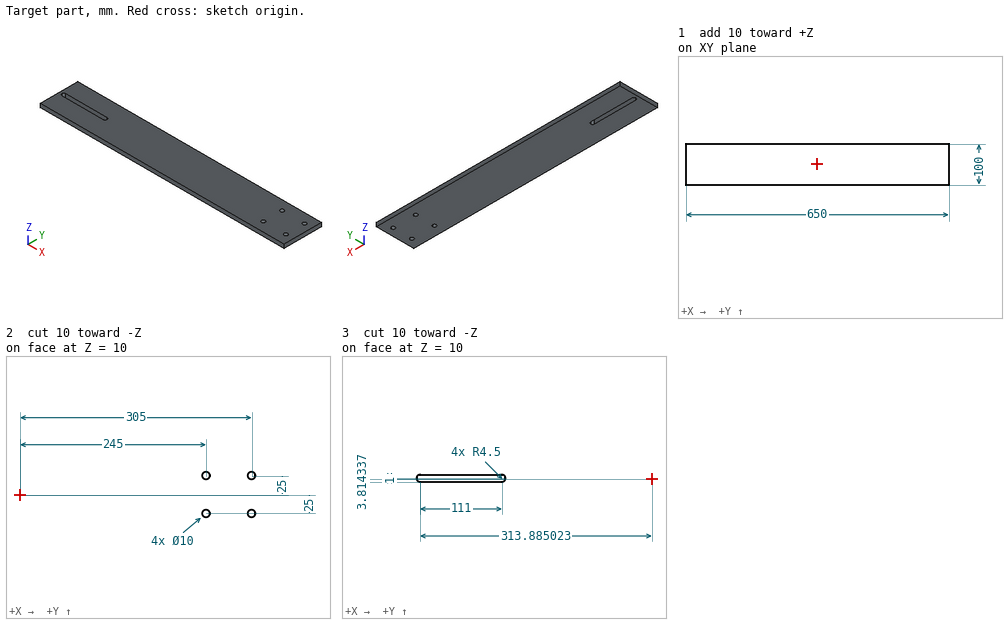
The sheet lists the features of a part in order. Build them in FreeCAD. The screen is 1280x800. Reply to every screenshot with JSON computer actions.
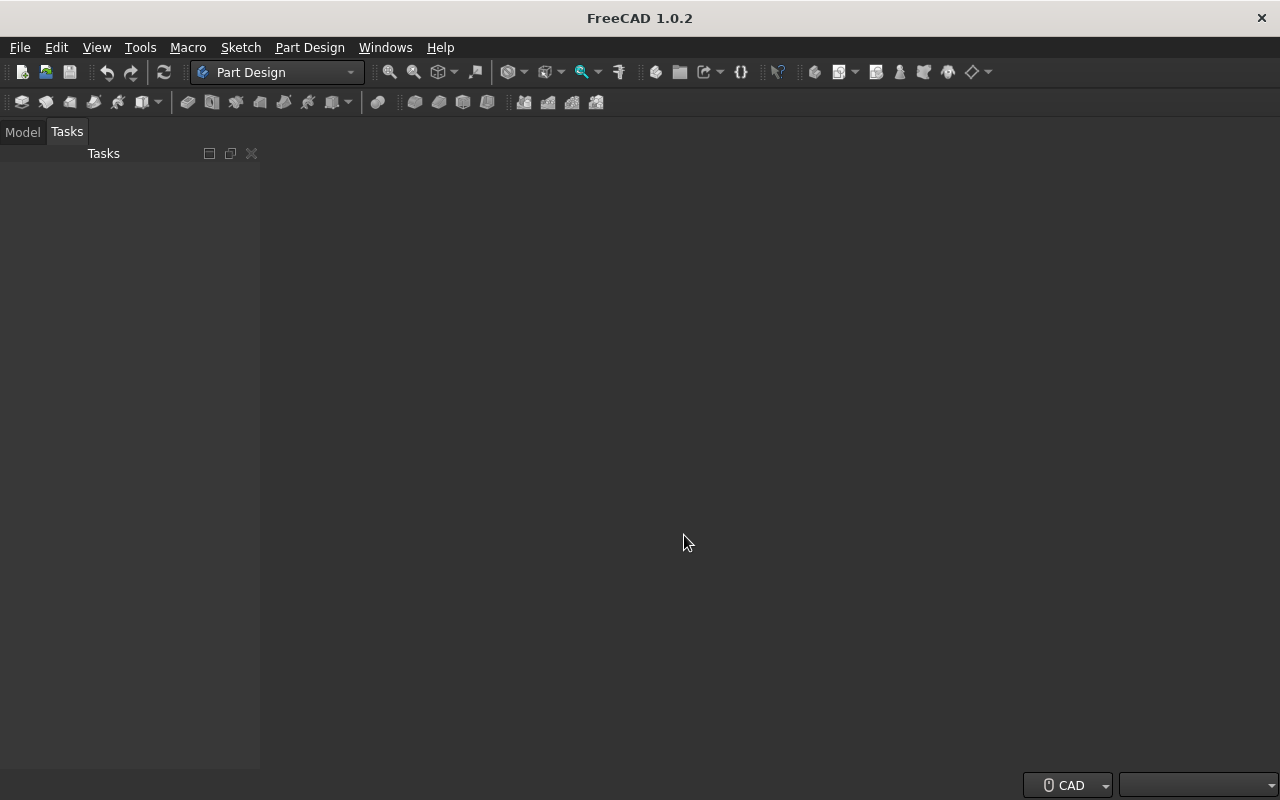
{"action": "key", "text": "ctrl+n"}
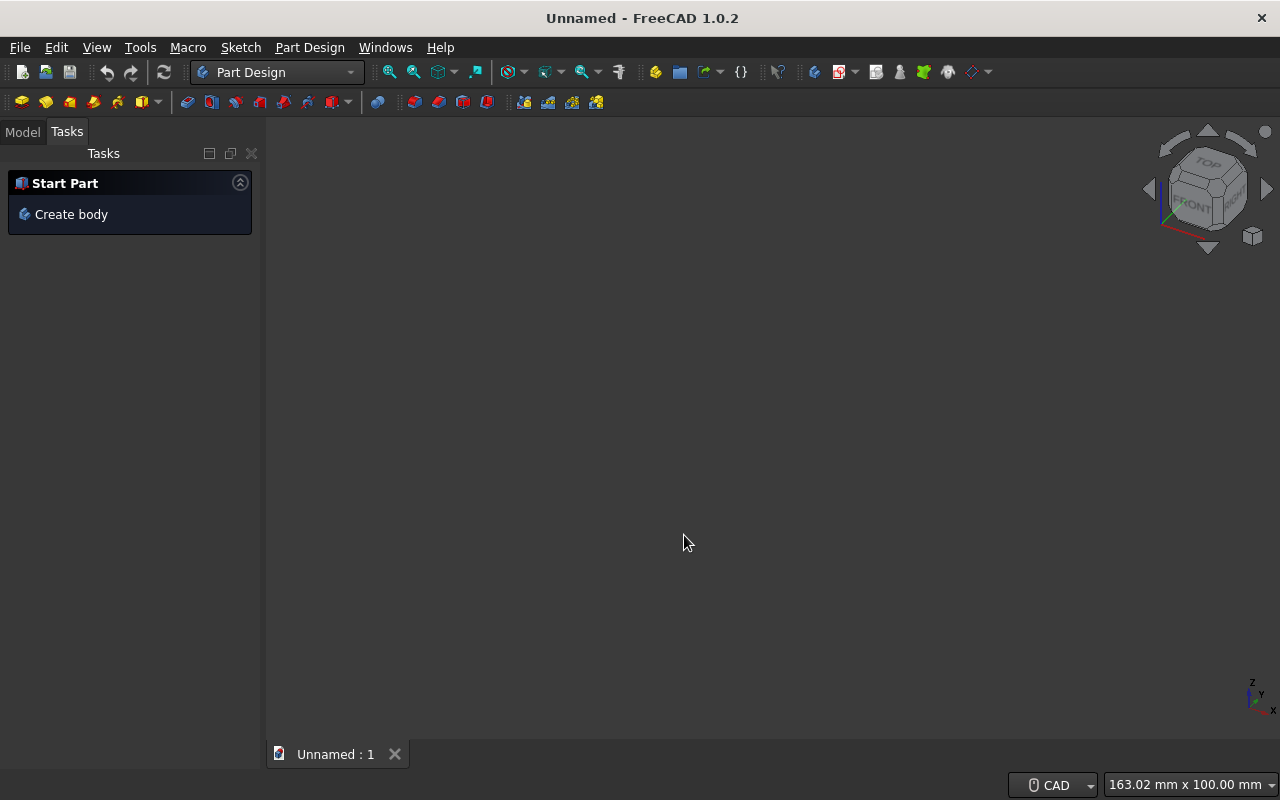
{"action": "left_click", "coordinate": [840, 72]}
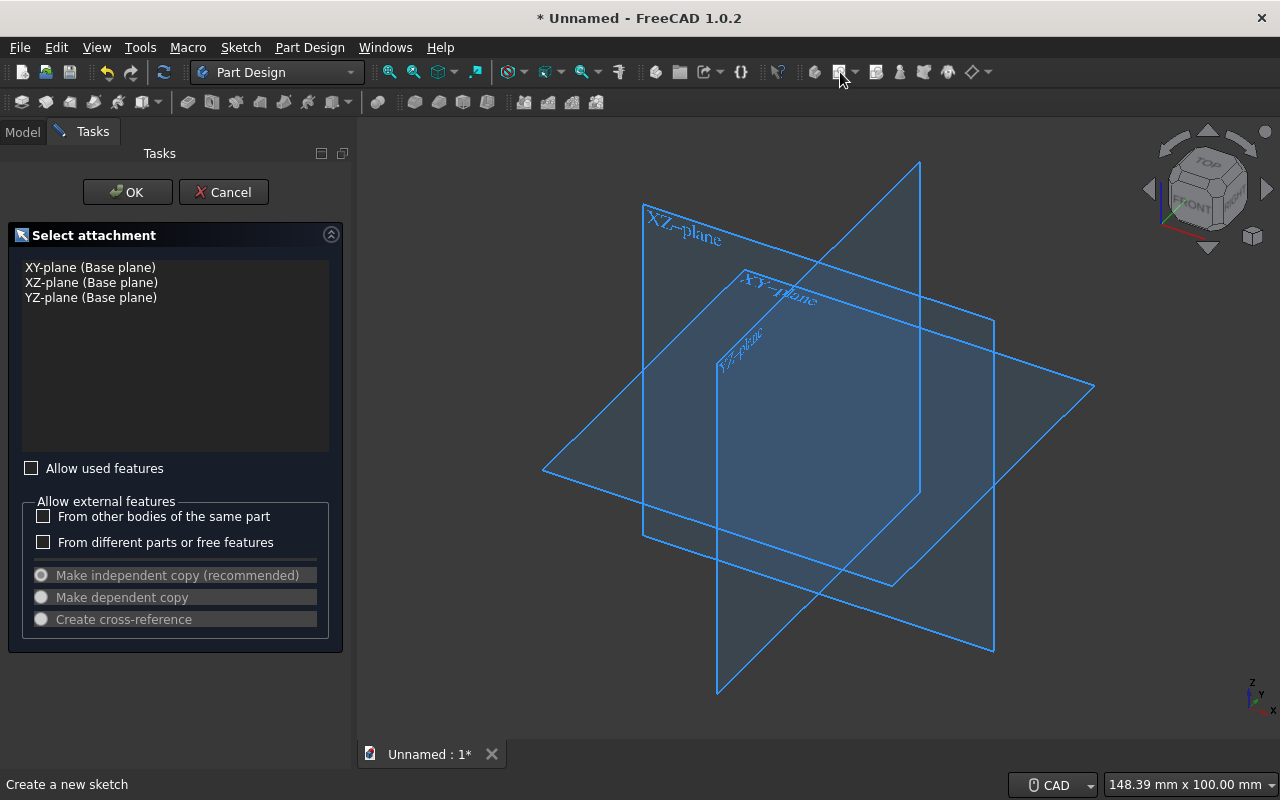
{"action": "left_click", "coordinate": [82, 268]}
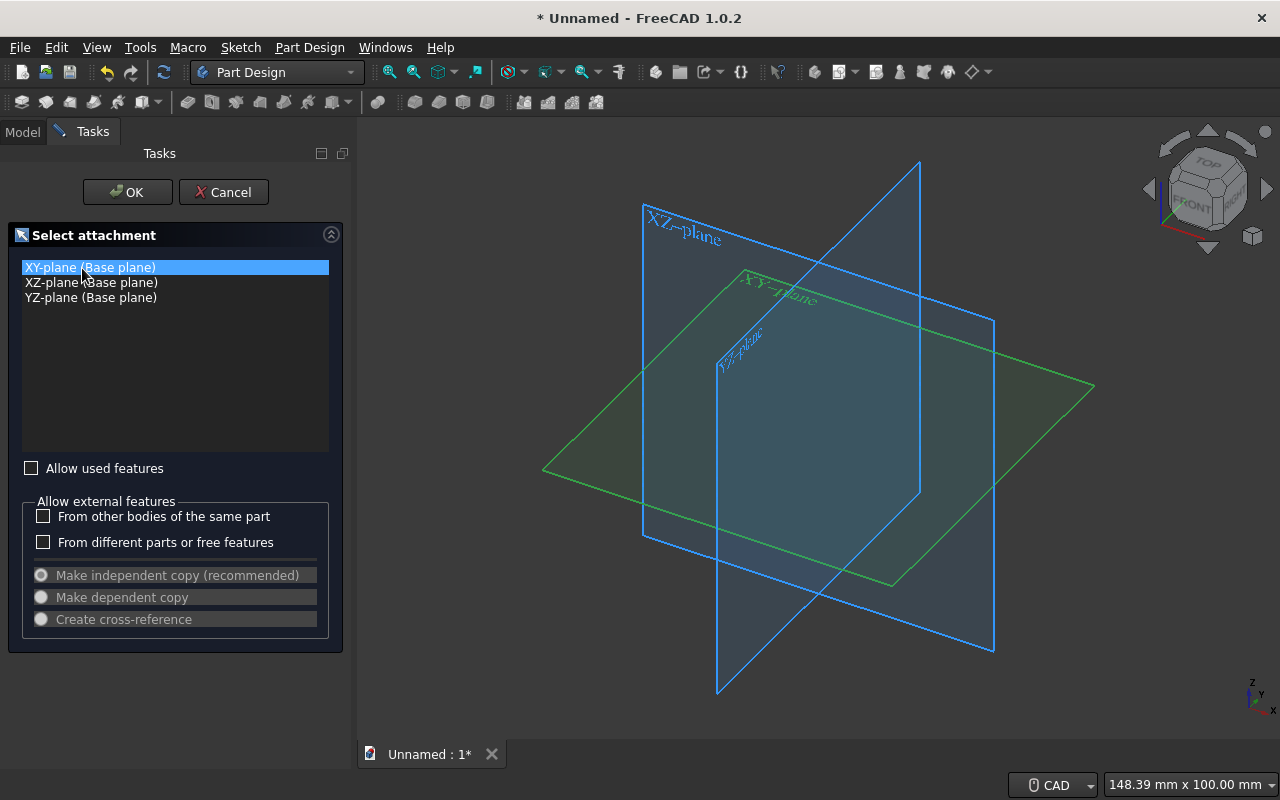
{"action": "left_click", "coordinate": [128, 192]}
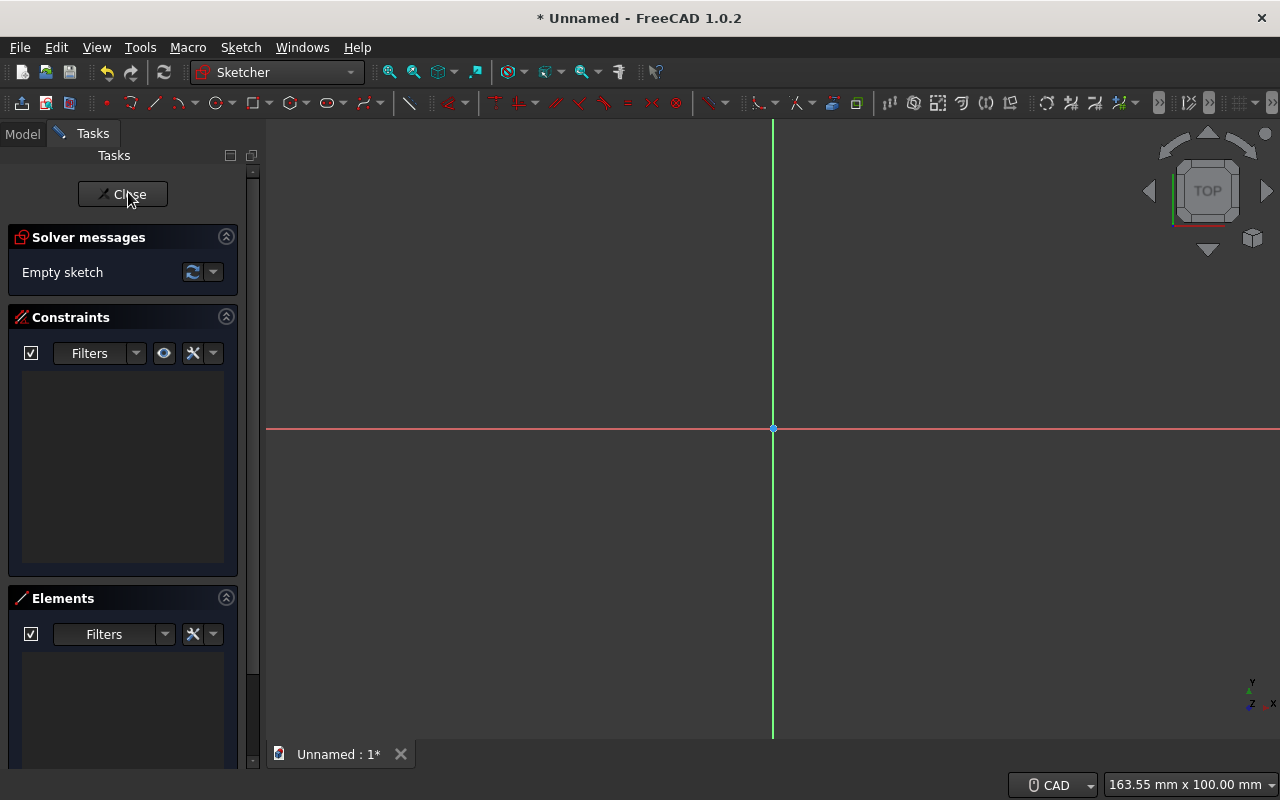
{"action": "scroll", "coordinate": [694, 429], "scroll_direction": "down", "scroll_amount": 10}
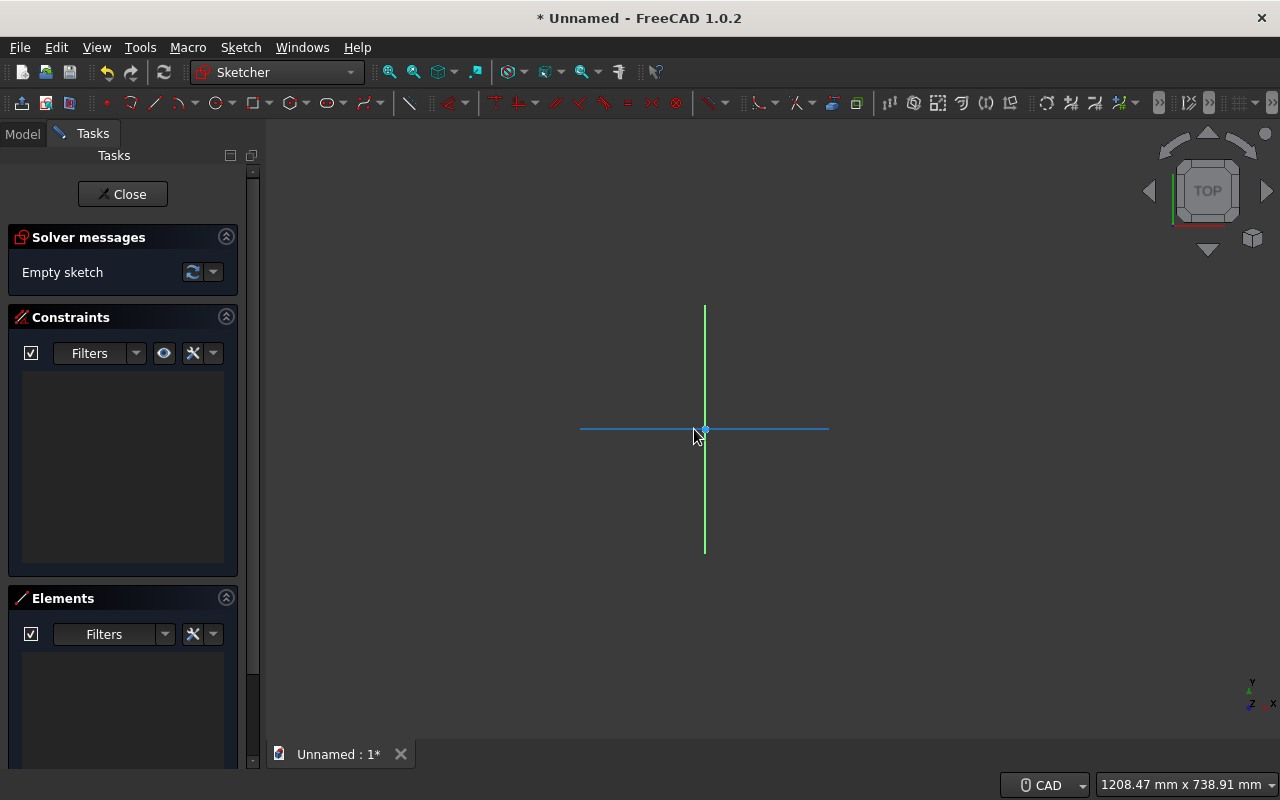
{"action": "left_click", "coordinate": [272, 104]}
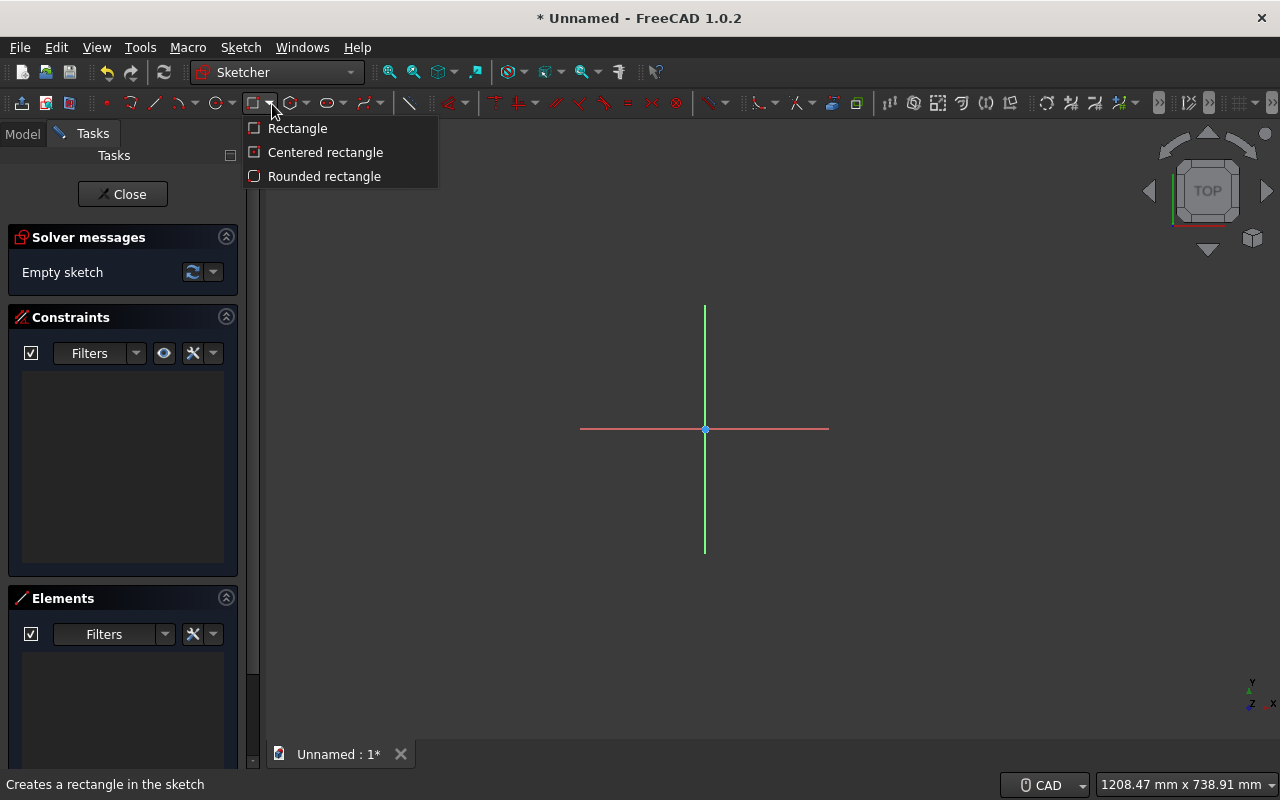
{"action": "left_click", "coordinate": [340, 152]}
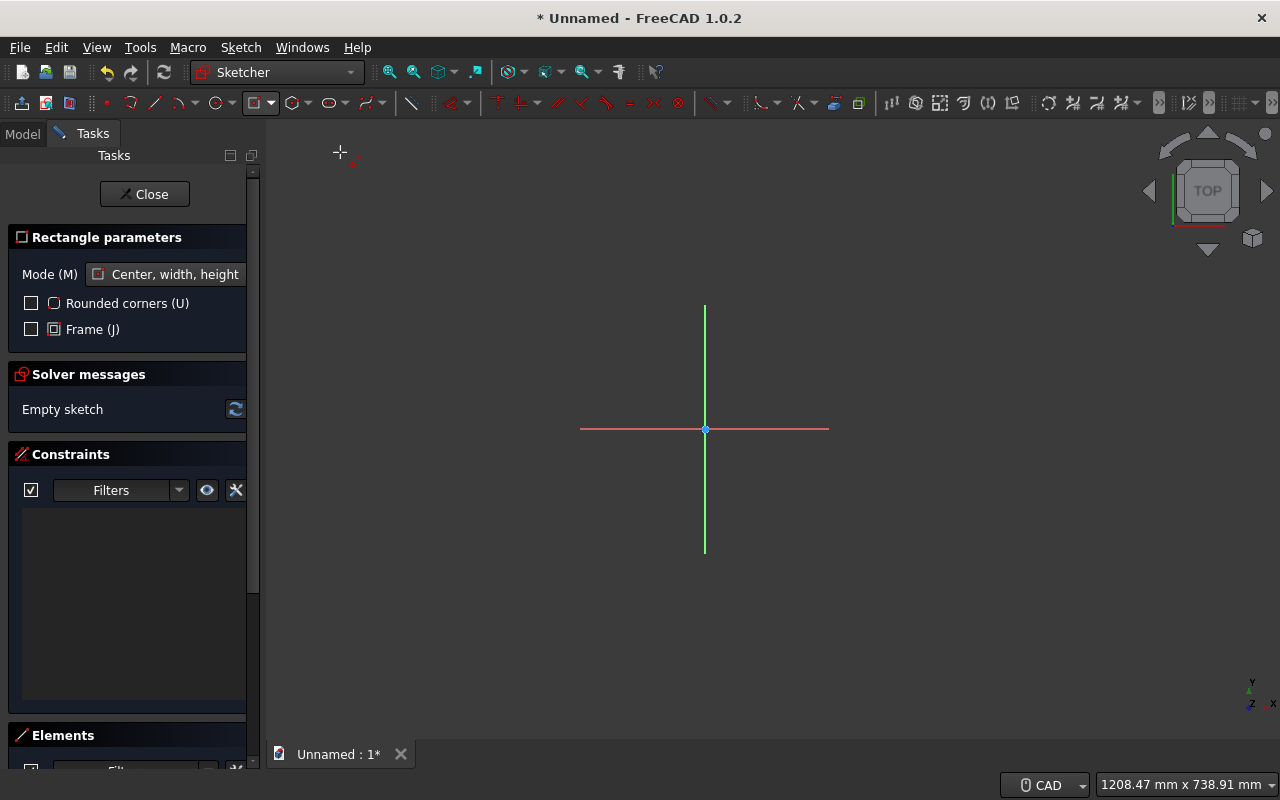
{"action": "left_click", "coordinate": [705, 429]}
{"action": "mouse_move", "coordinate": [978, 387]}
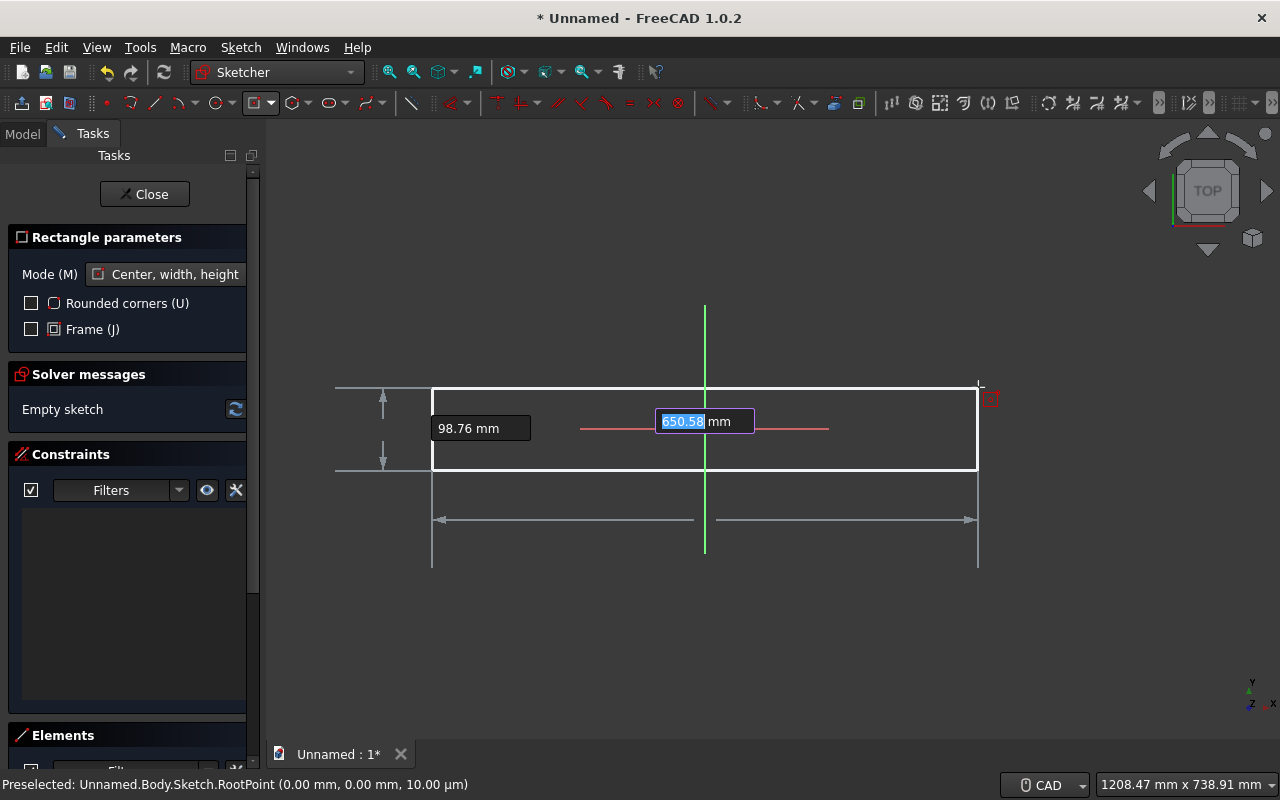
{"action": "type", "text": "650"}
{"action": "key", "text": "Tab"}
{"action": "type", "text": "100"}
{"action": "key", "text": "Return"}
{"action": "key", "text": "Escape"}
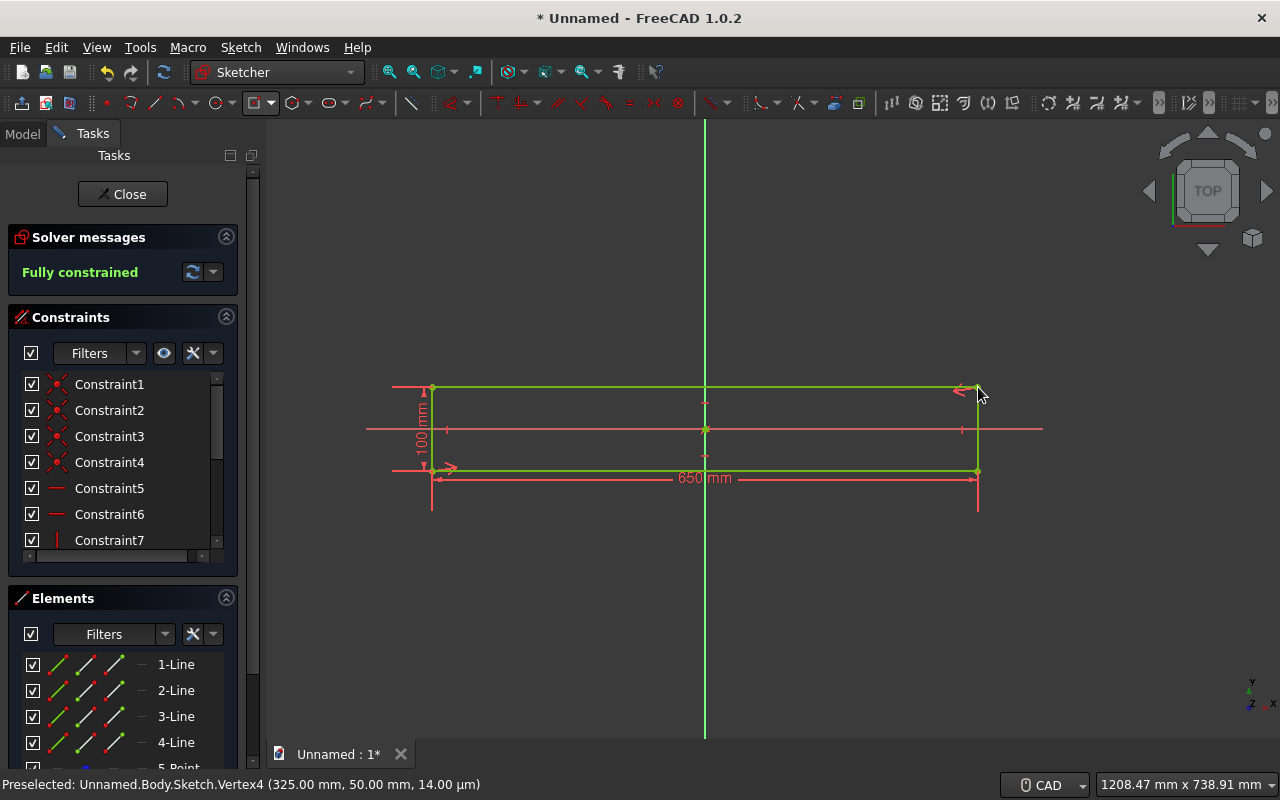
{"action": "left_click", "coordinate": [123, 194]}